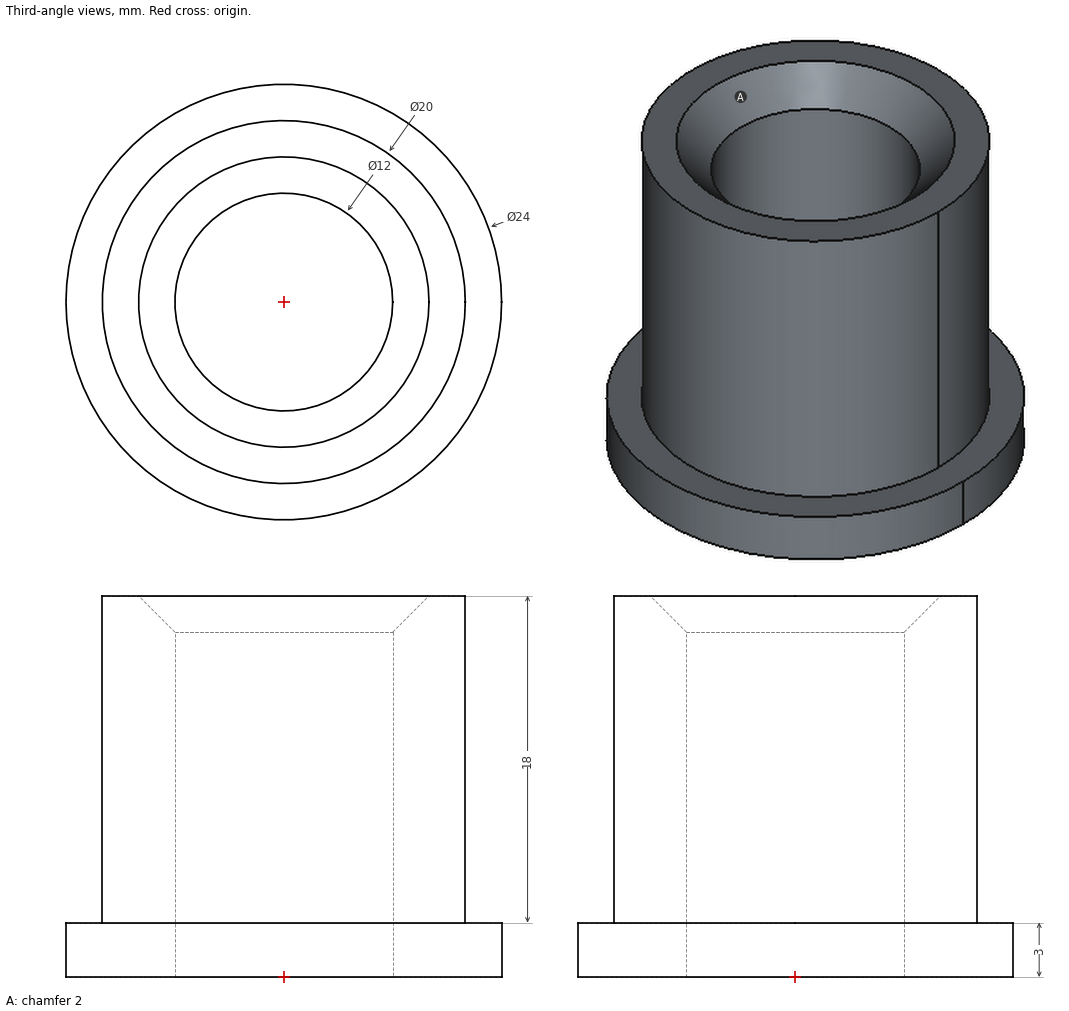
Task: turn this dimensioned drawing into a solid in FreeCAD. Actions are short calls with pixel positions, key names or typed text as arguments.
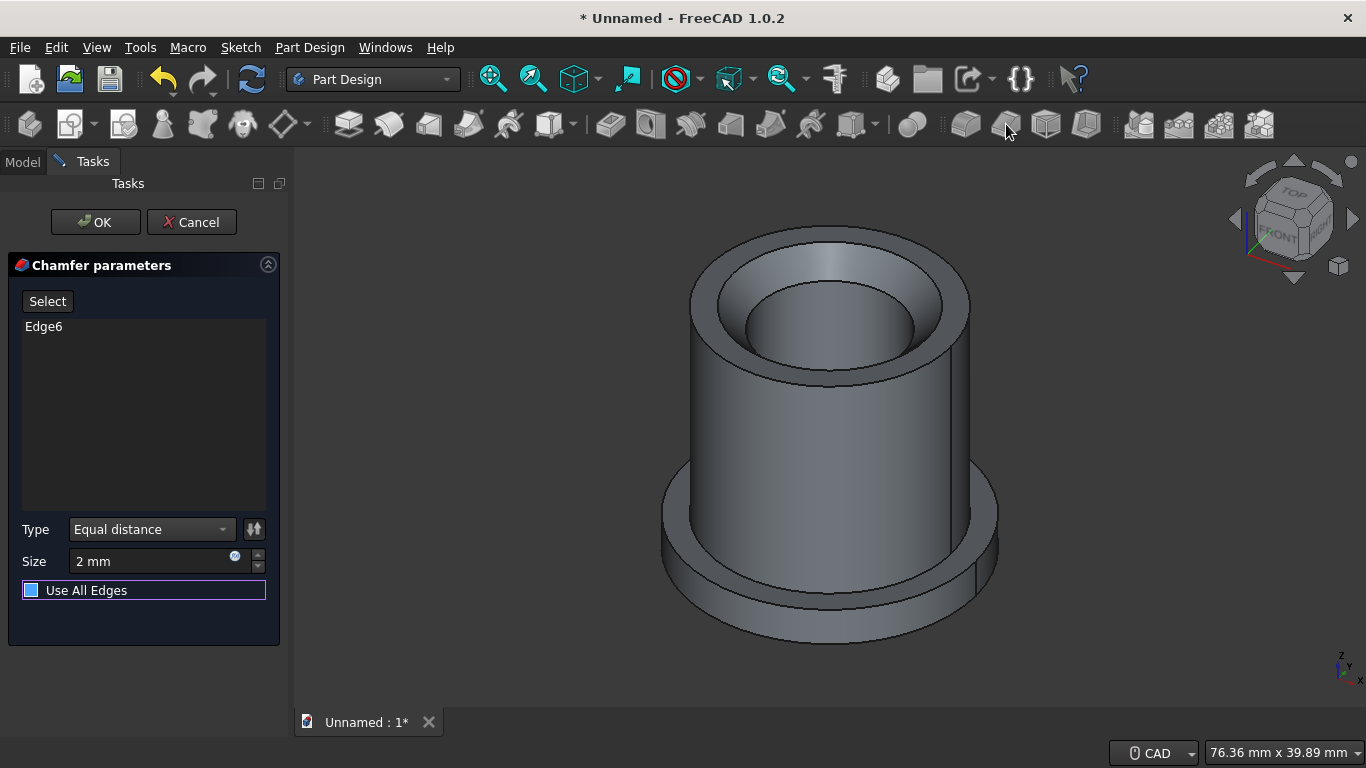
click(96, 222)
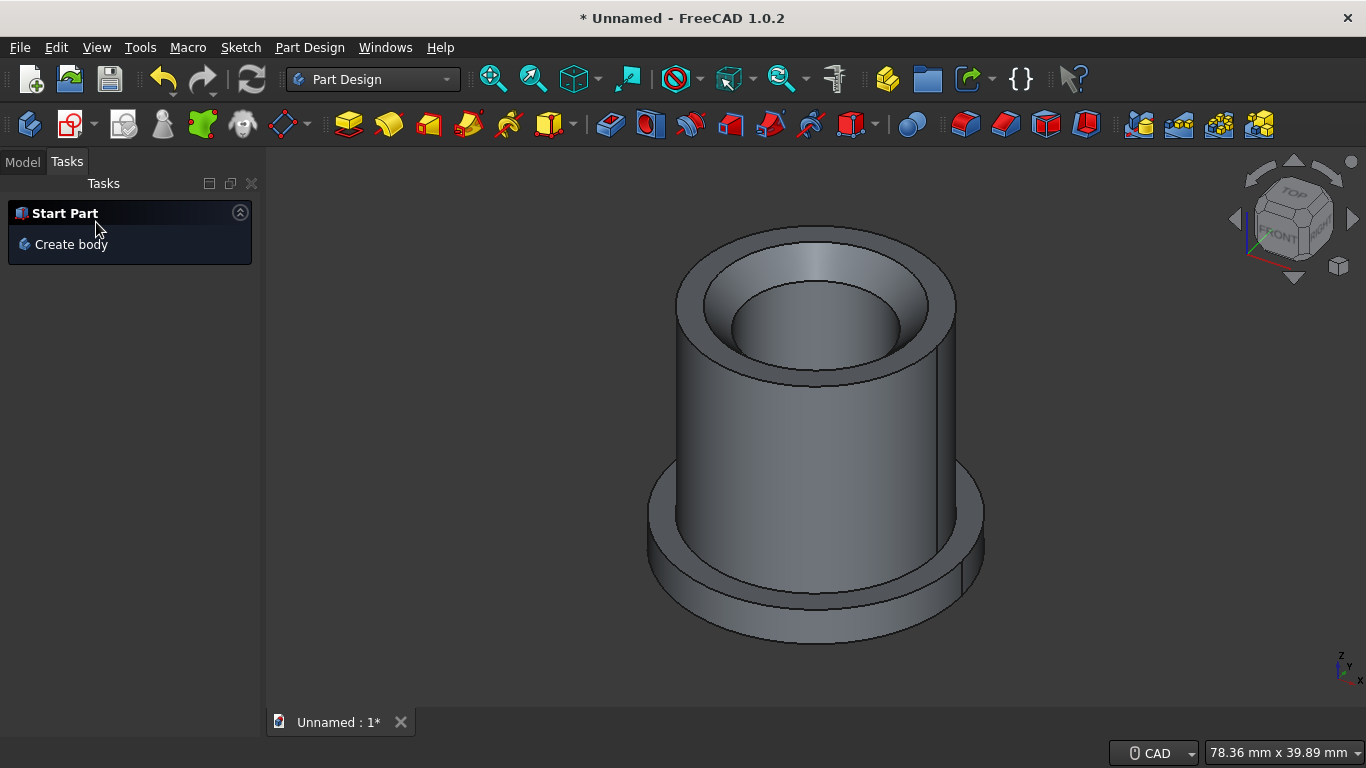
key(0)